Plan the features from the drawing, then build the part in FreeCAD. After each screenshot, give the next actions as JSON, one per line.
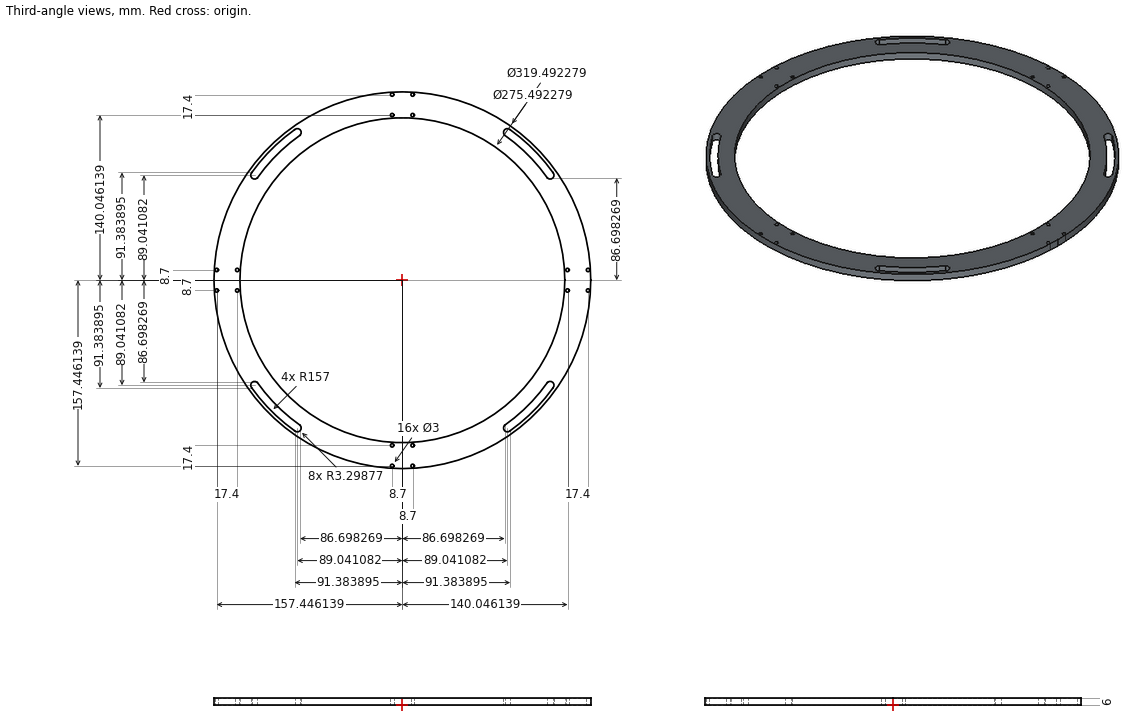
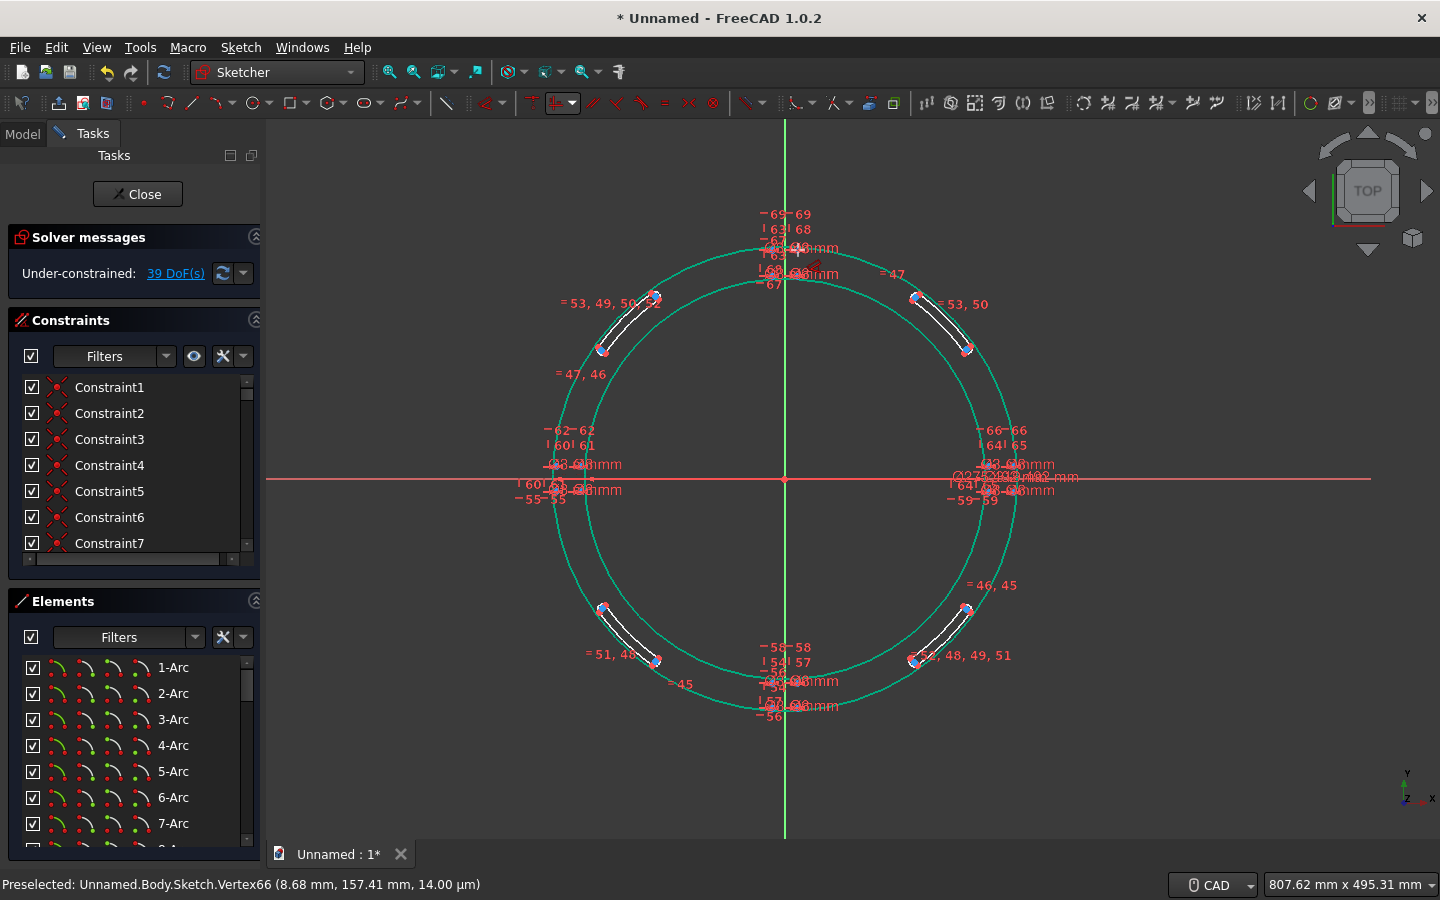
{"action": "scroll", "coordinate": [656, 666], "scroll_direction": "up", "scroll_amount": 11}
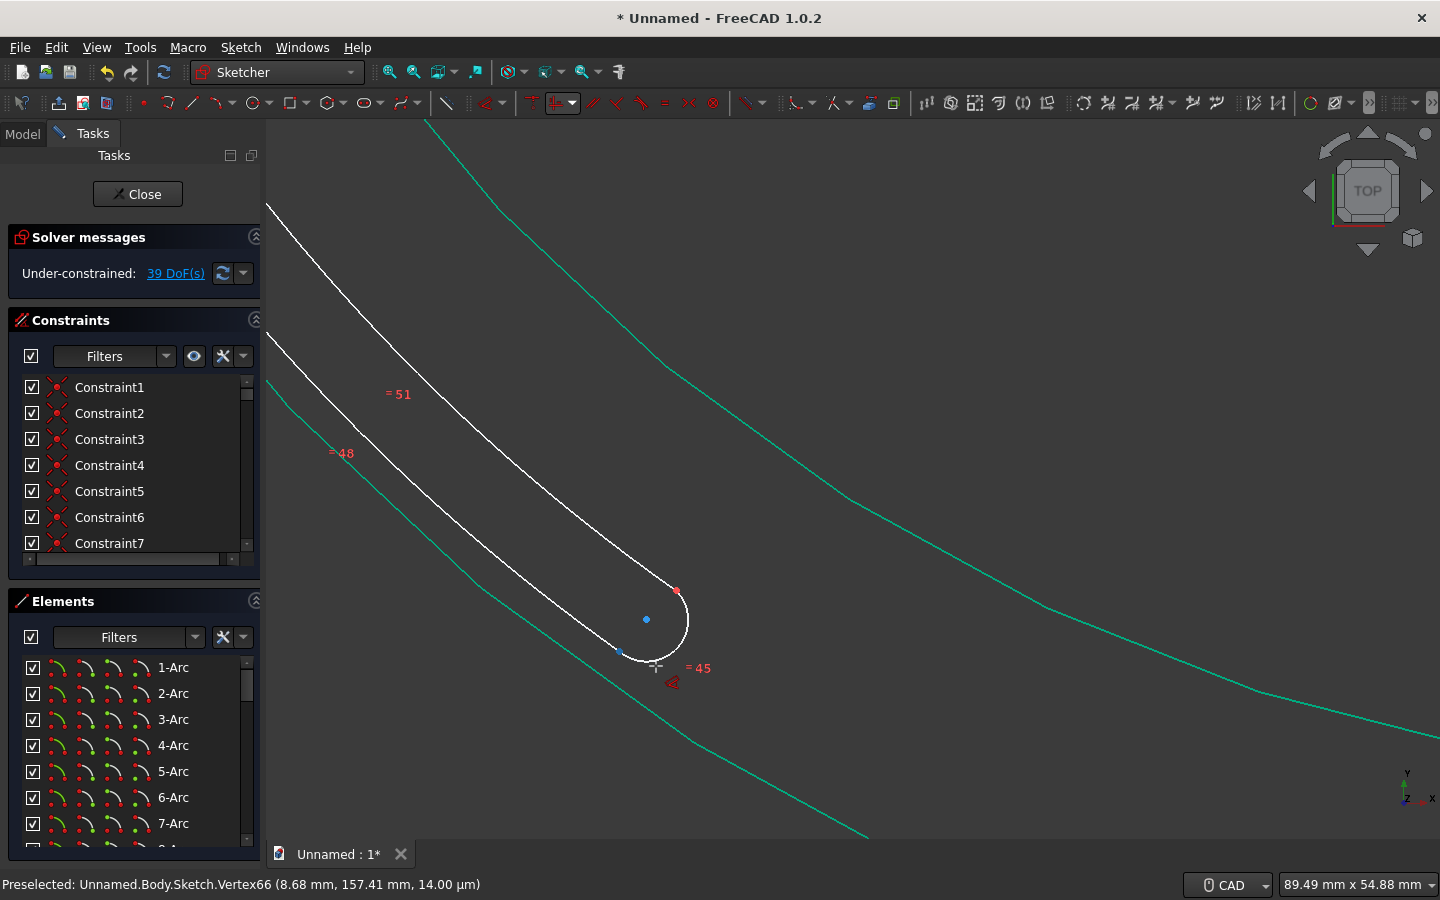
{"action": "left_click", "coordinate": [655, 661]}
{"action": "left_click", "coordinate": [661, 692]}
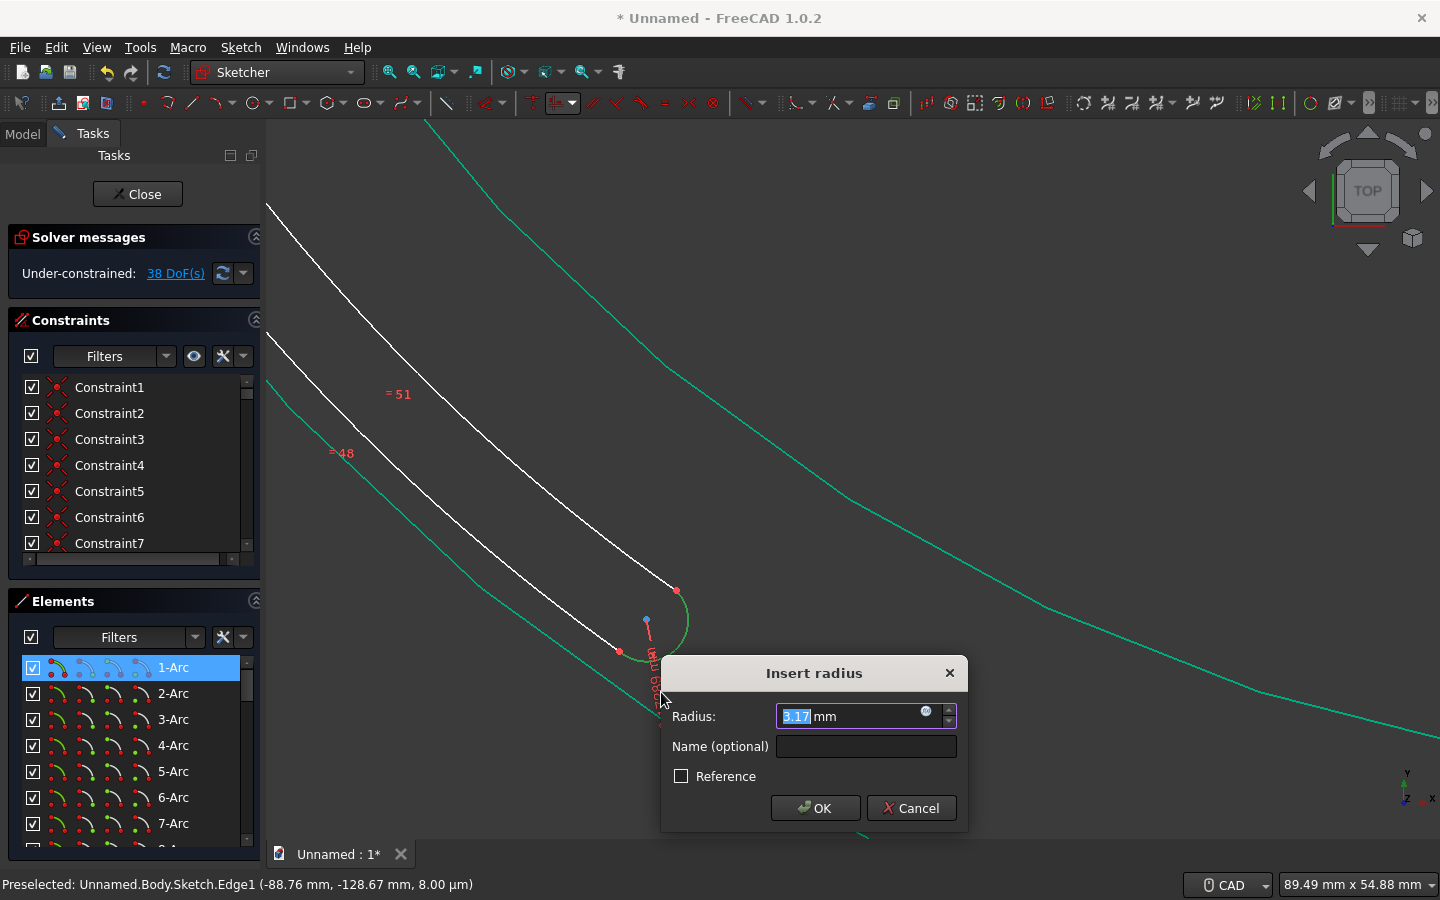
{"action": "type", "text": "3.29877"}
{"action": "key", "text": "Return"}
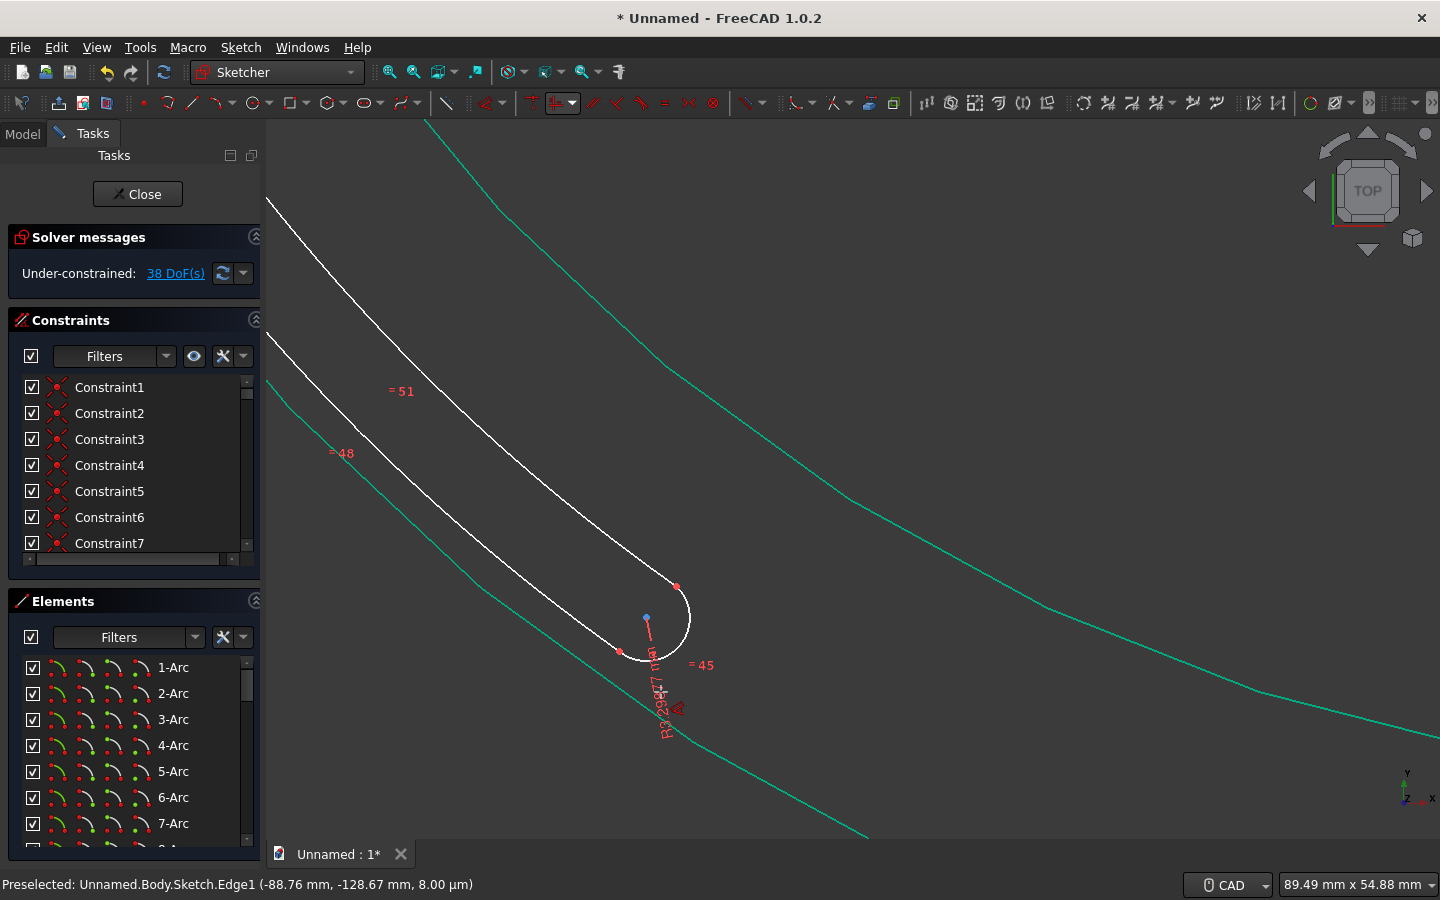
{"action": "left_click", "coordinate": [460, 525]}
{"action": "left_click", "coordinate": [424, 566]}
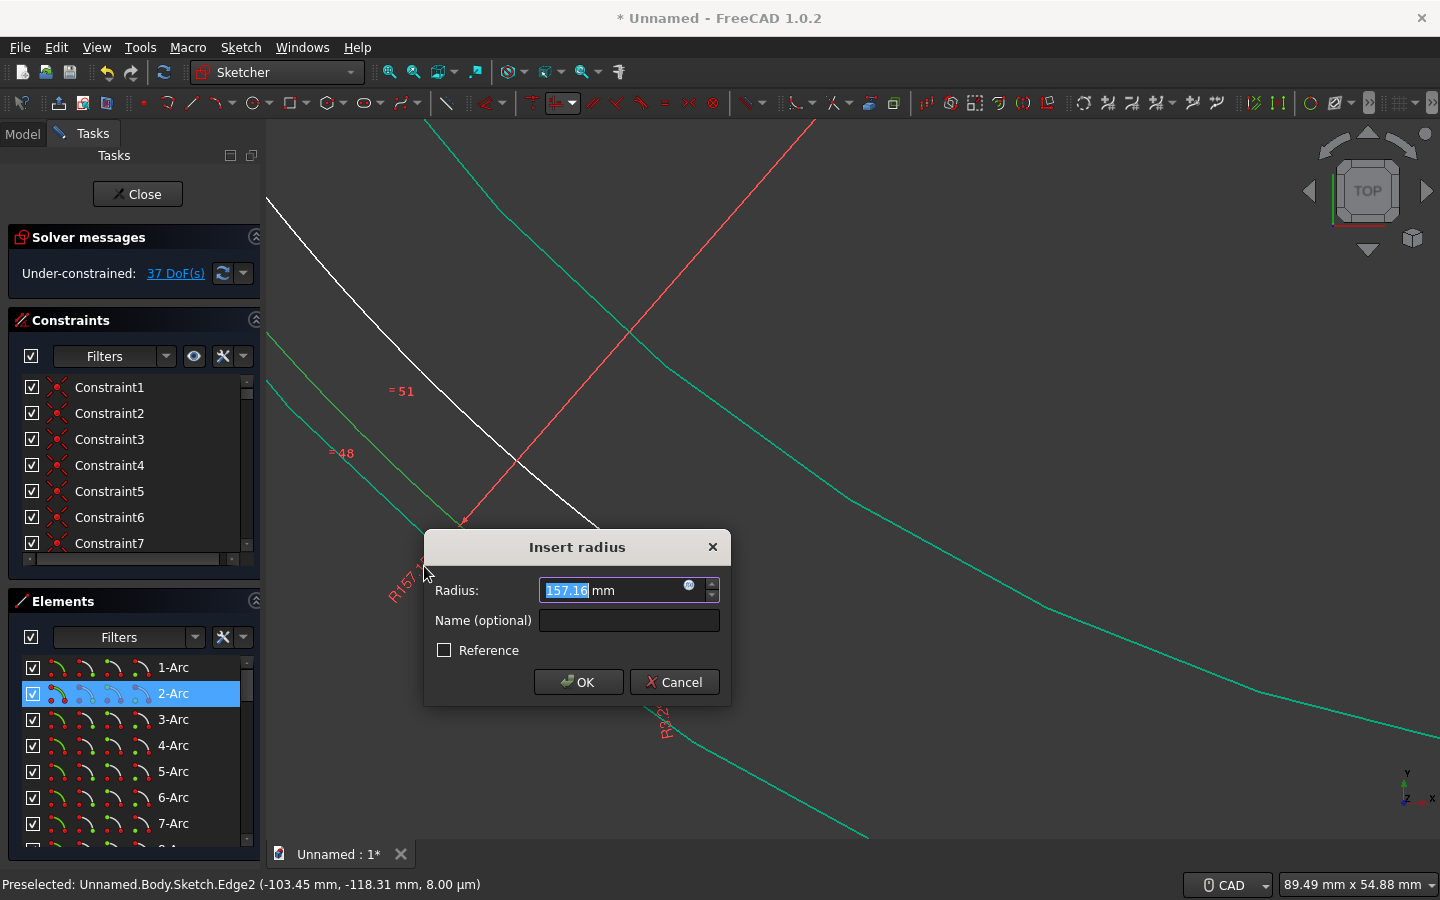
{"action": "type", "text": "157"}
{"action": "key", "text": "Return"}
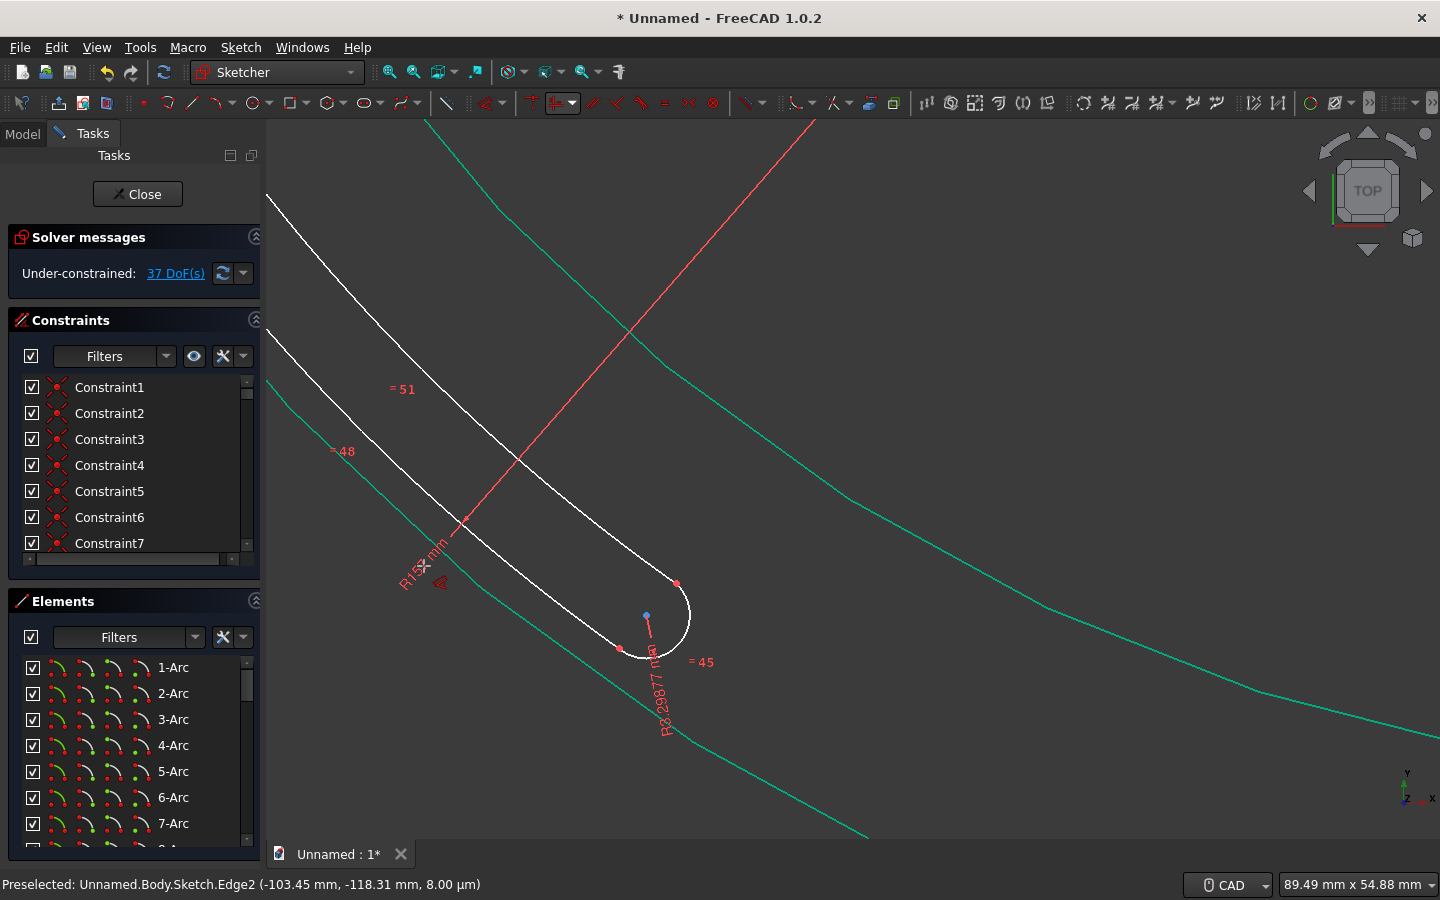
{"action": "scroll", "coordinate": [656, 667], "scroll_direction": "down", "scroll_amount": 11}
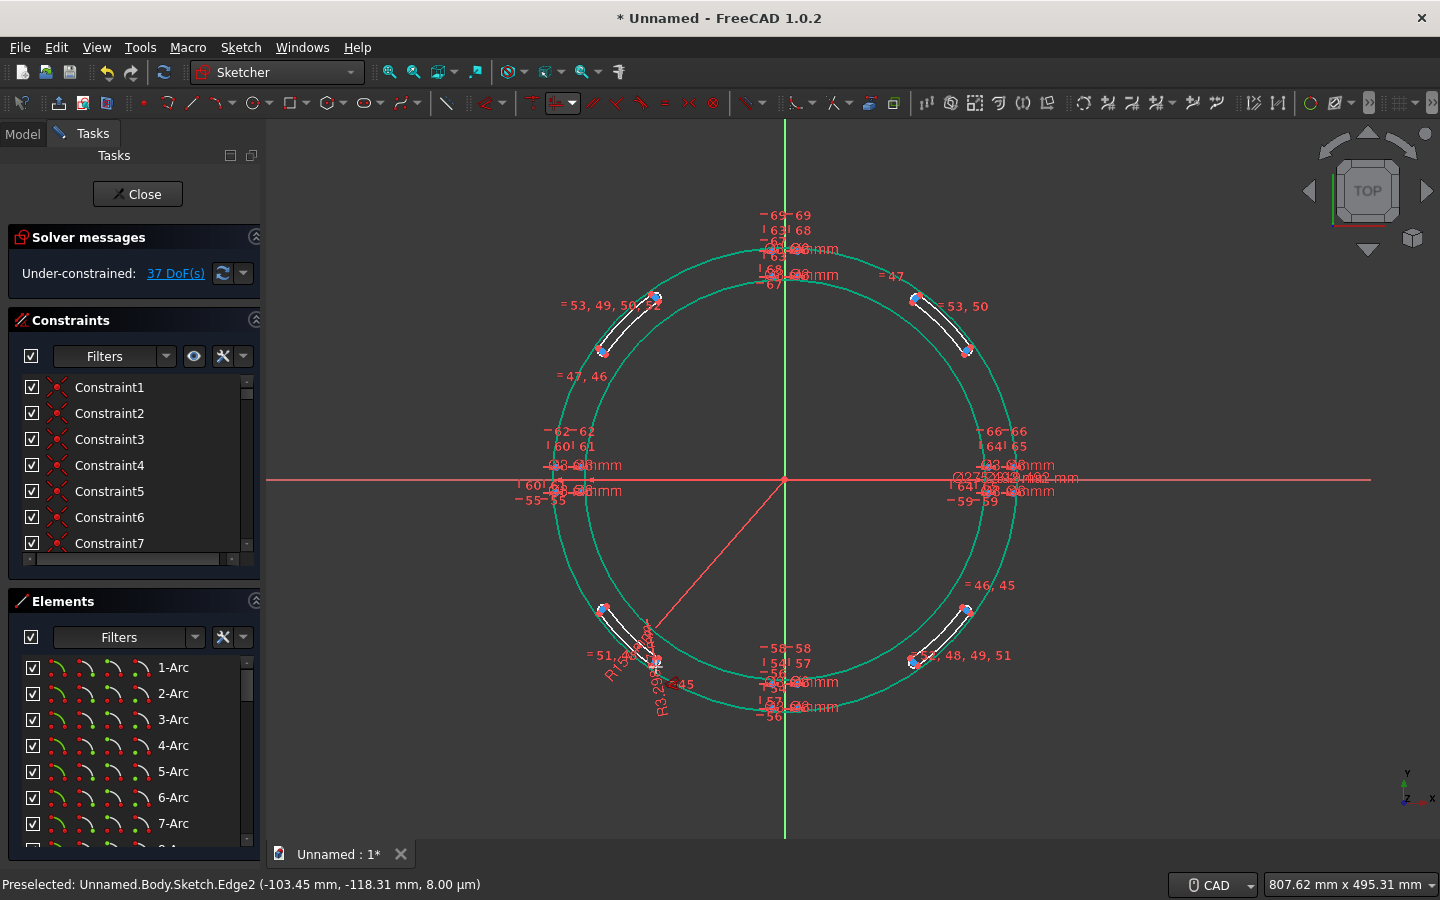
{"action": "scroll", "coordinate": [772, 709], "scroll_direction": "up", "scroll_amount": 6}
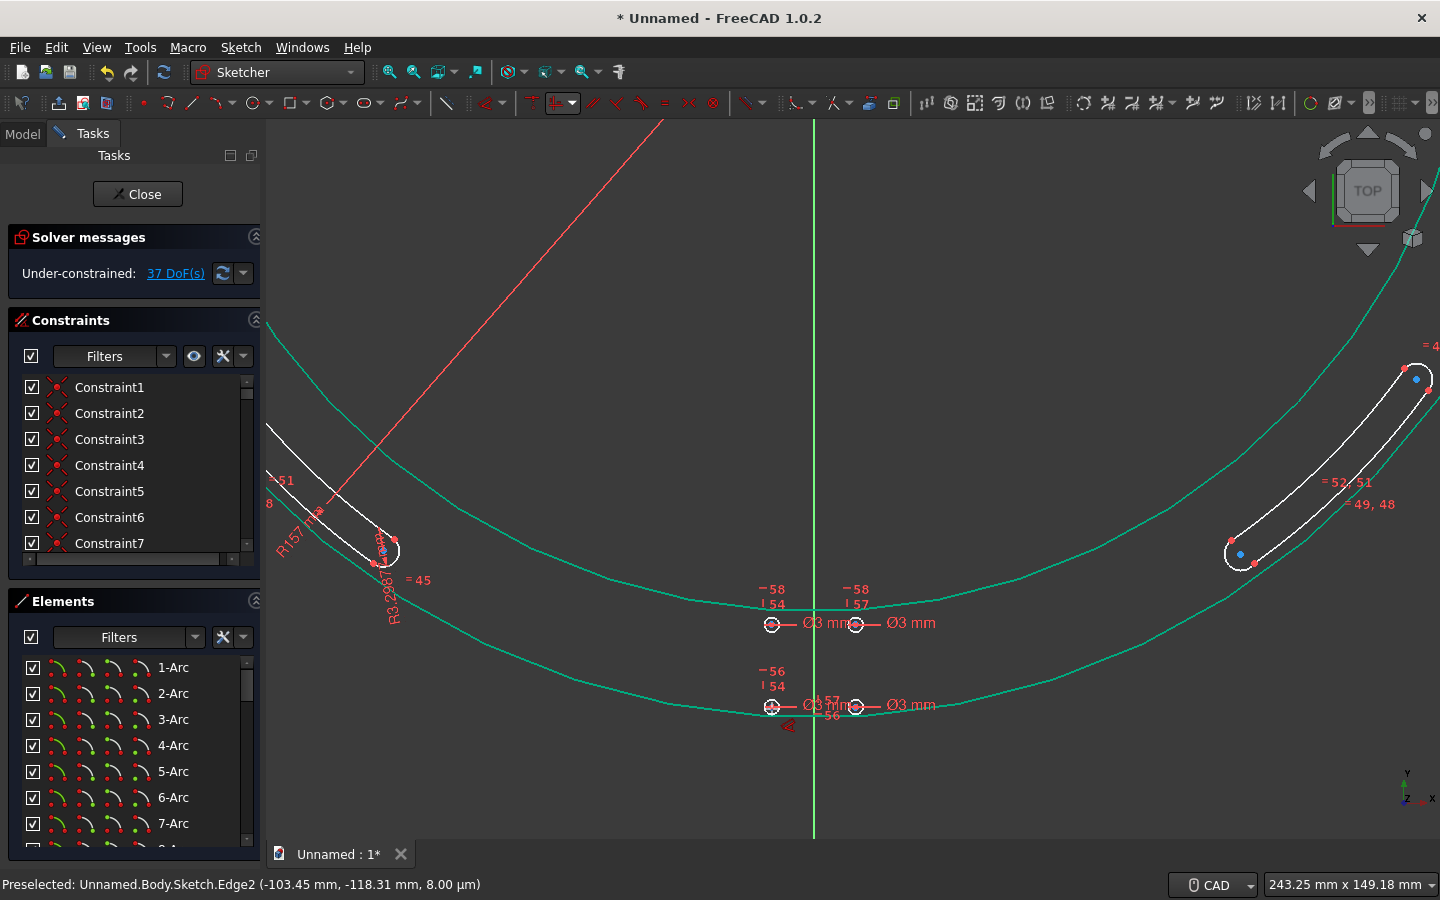
{"action": "left_click", "coordinate": [772, 707]}
{"action": "left_click", "coordinate": [793, 741]}